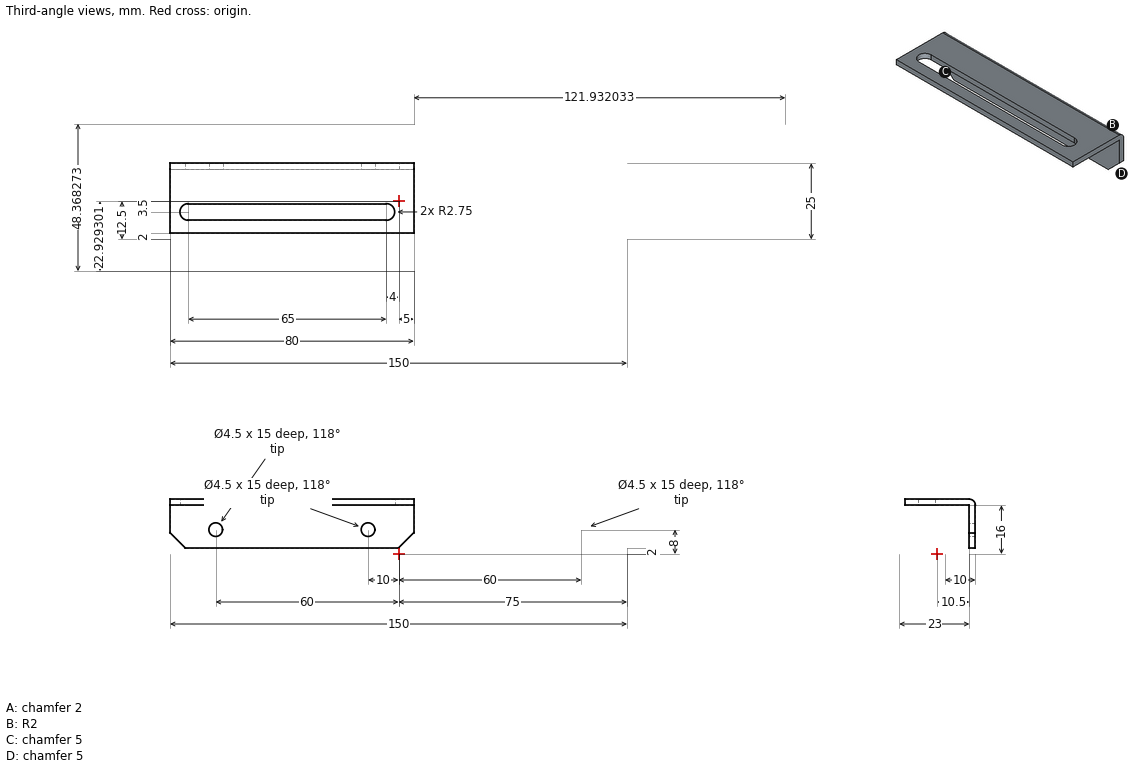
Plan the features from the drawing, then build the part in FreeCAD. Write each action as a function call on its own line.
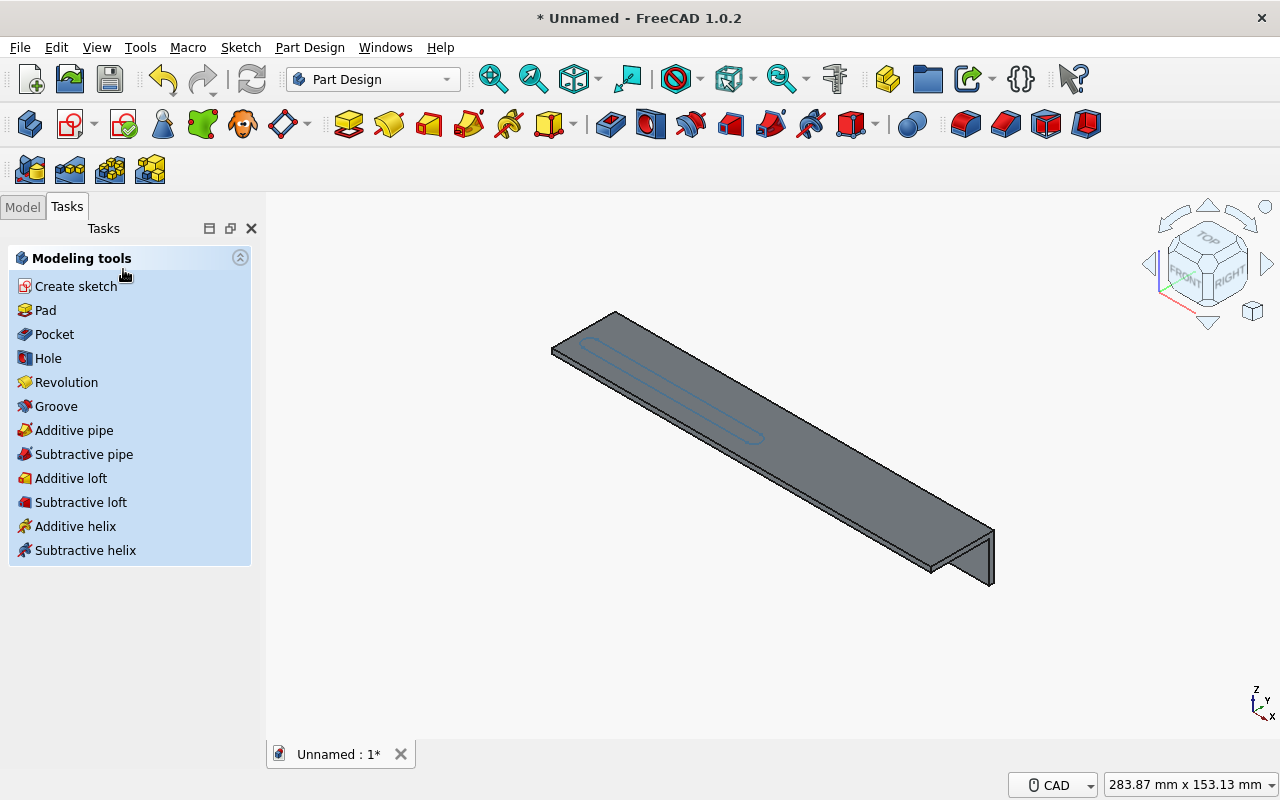
click(612, 124)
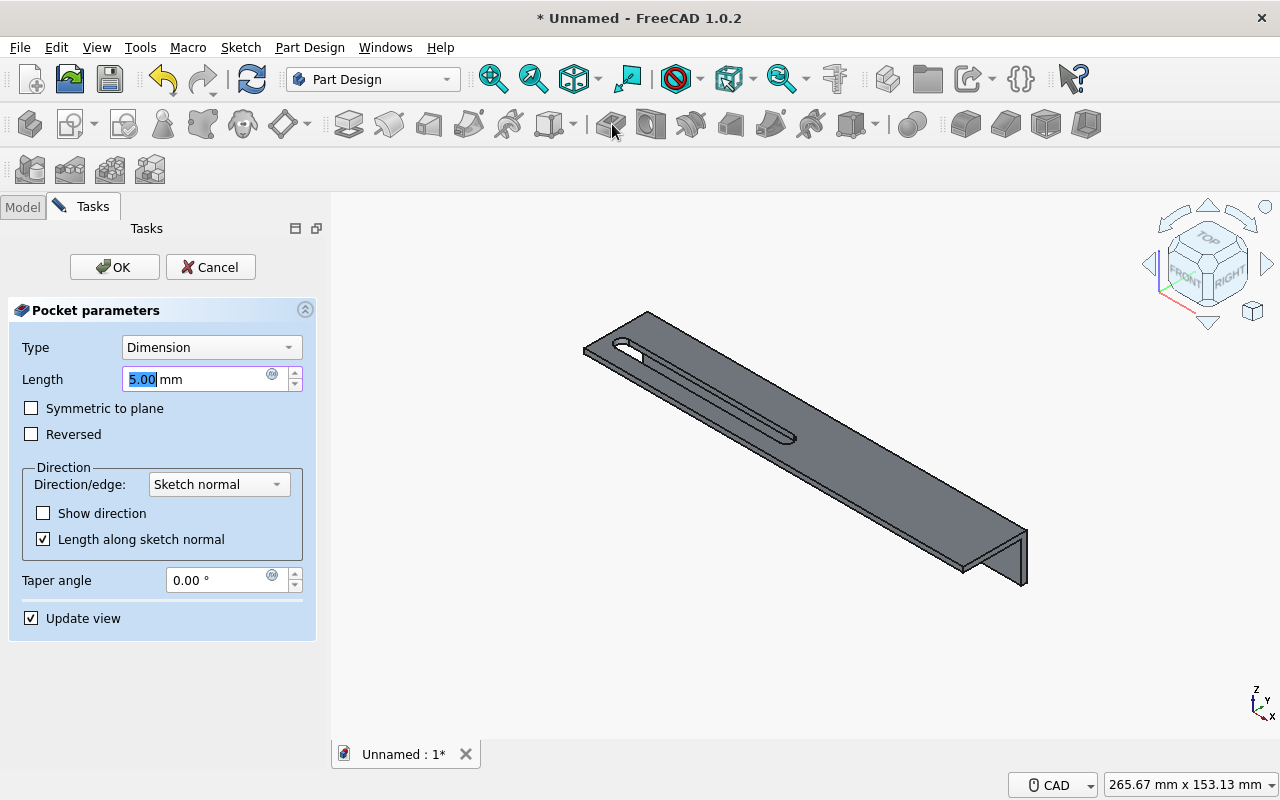
click(212, 348)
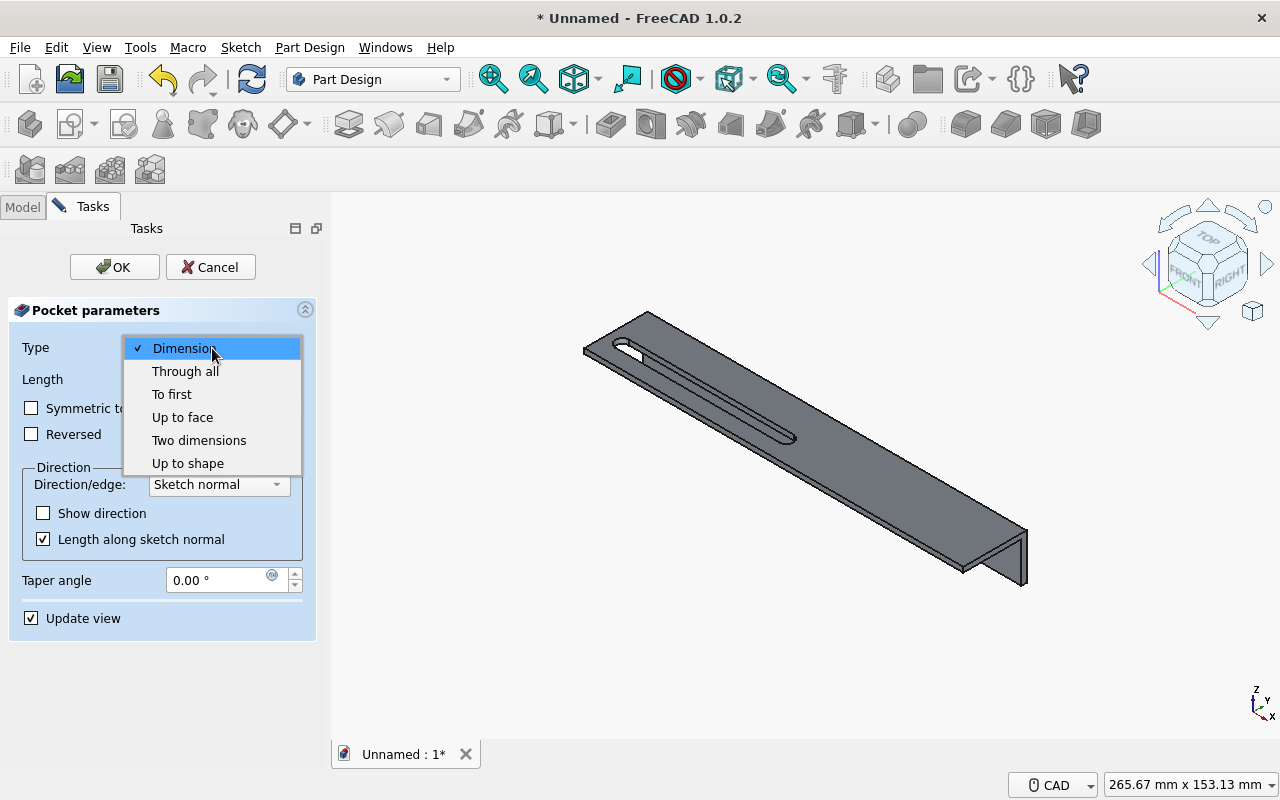
click(212, 372)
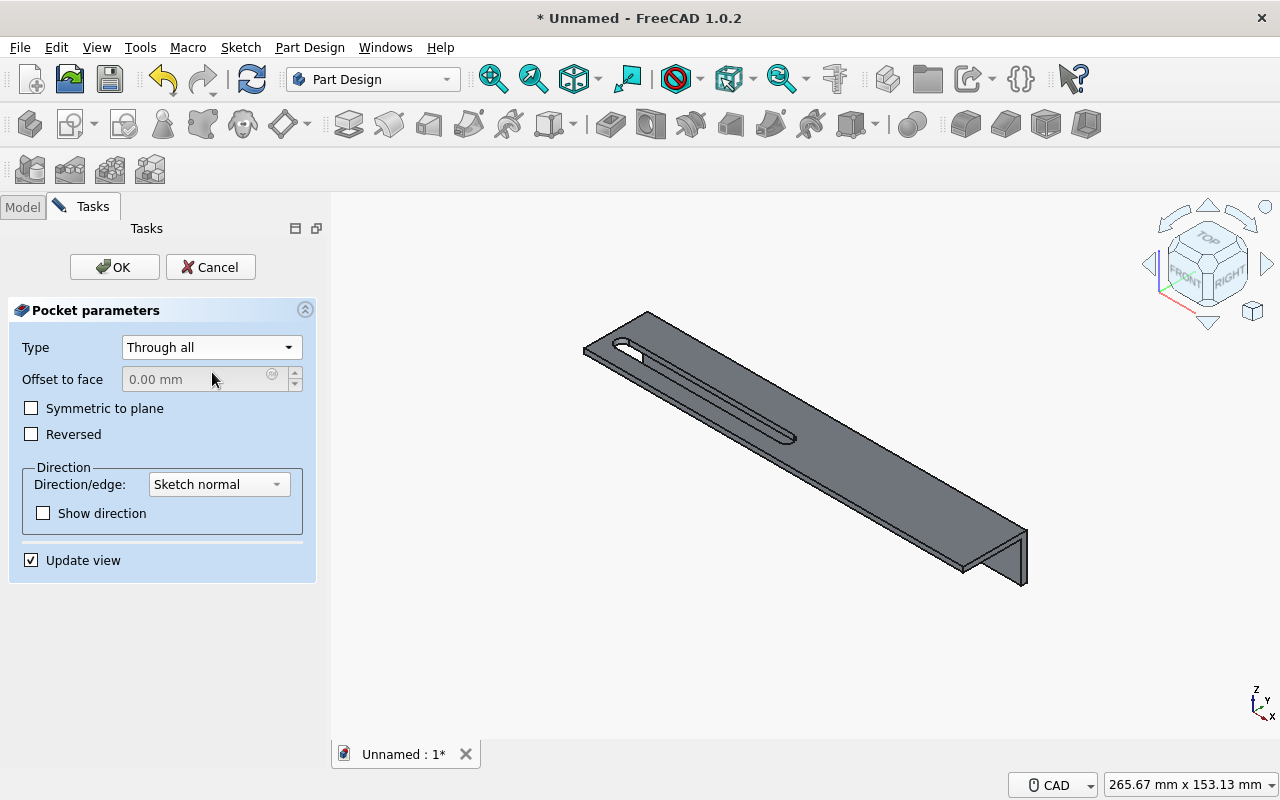
click(115, 267)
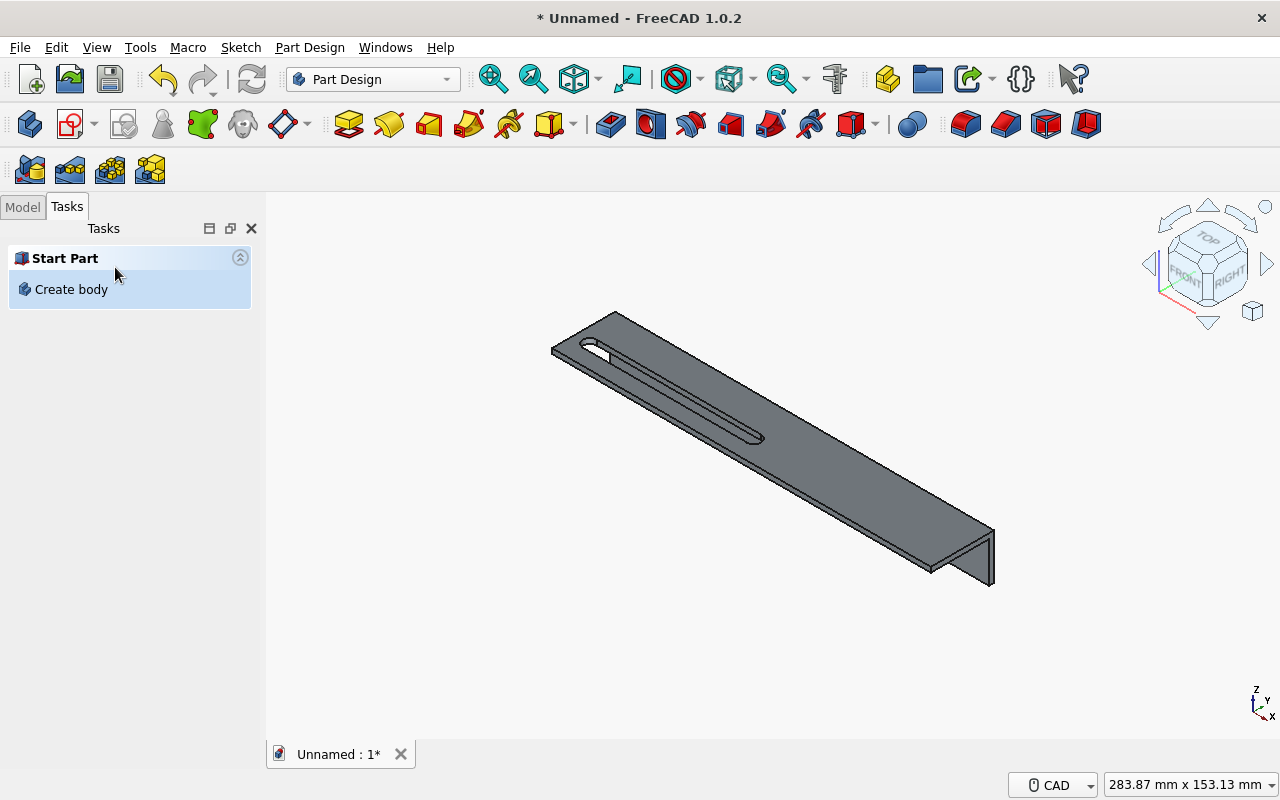
key(4)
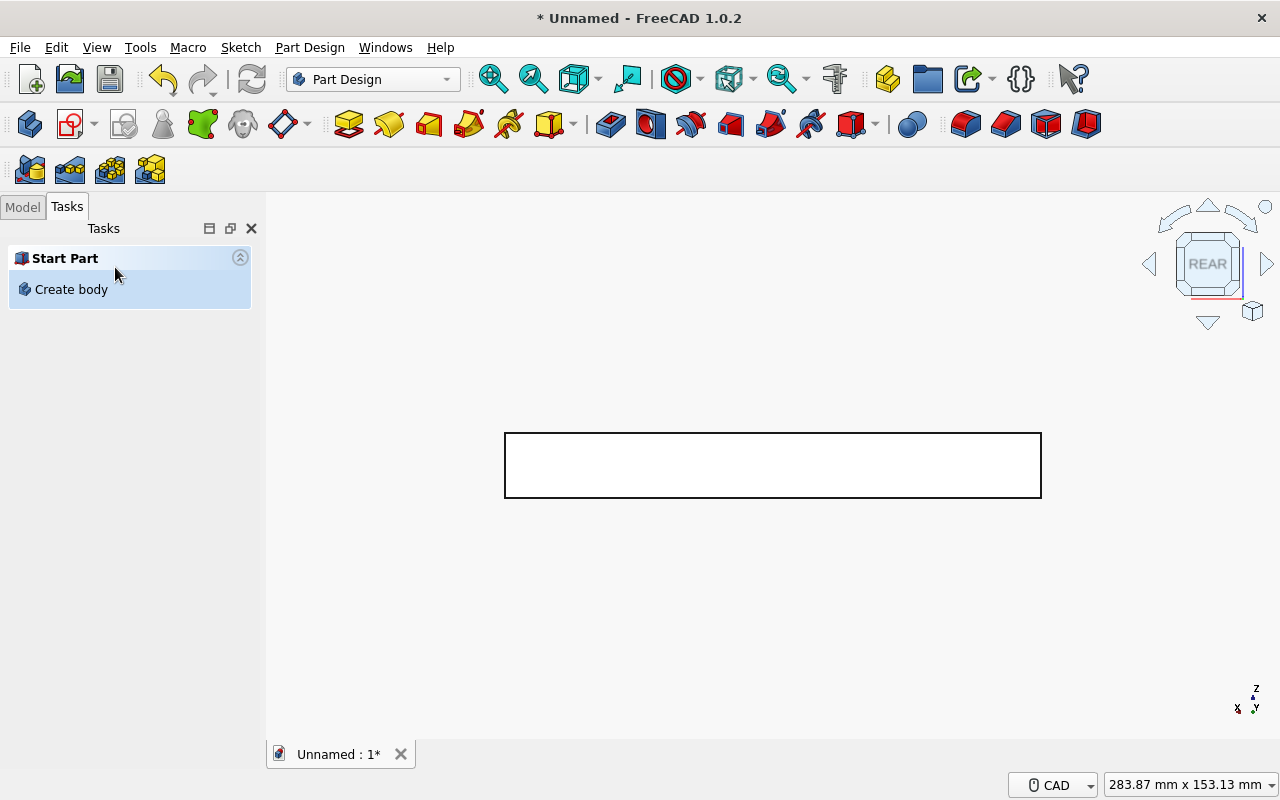
click(543, 465)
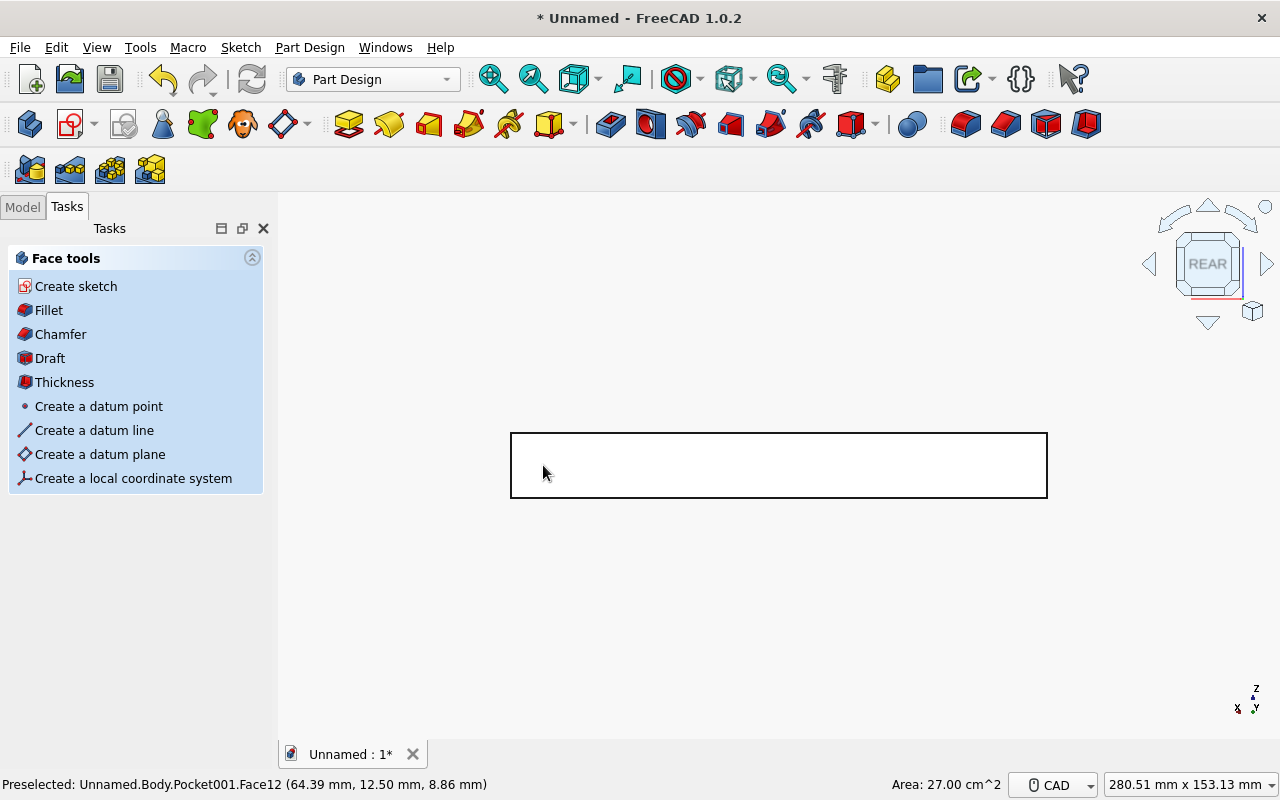
click(70, 124)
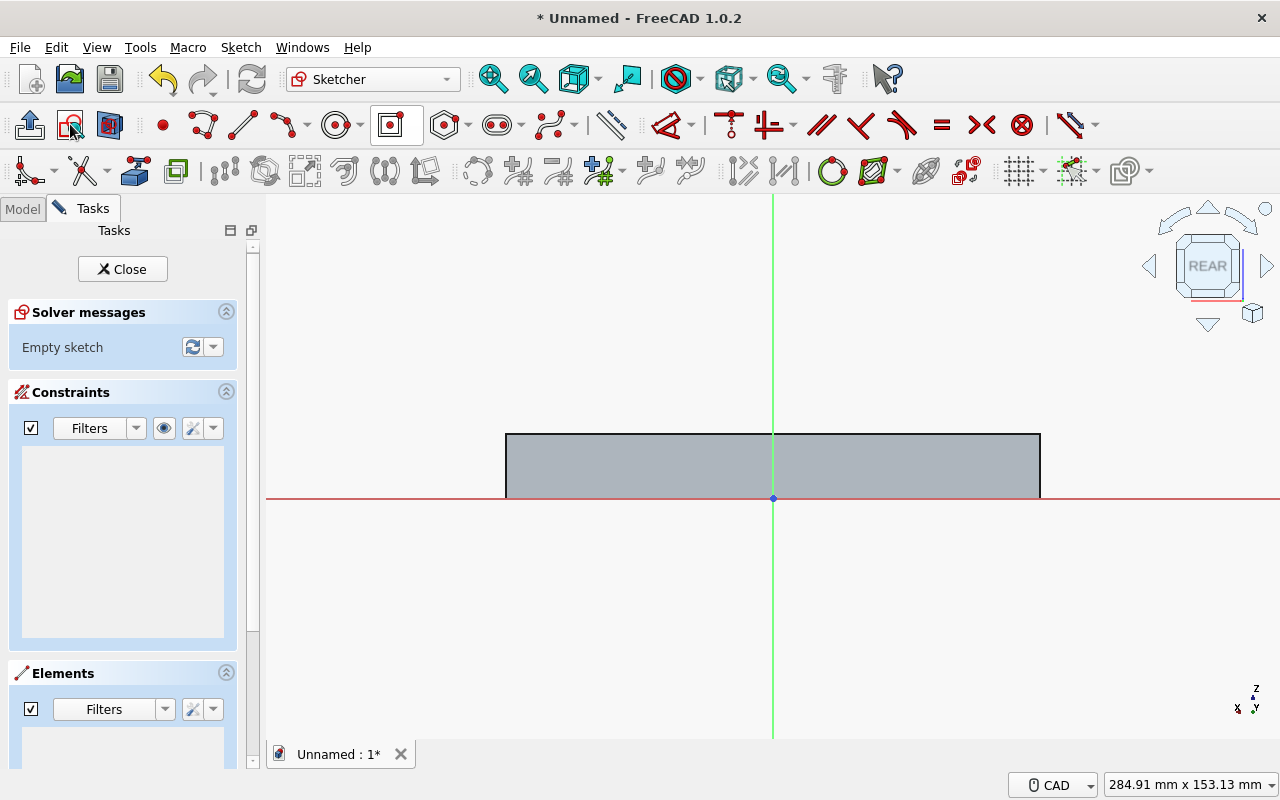
scroll(552, 470, up, 15)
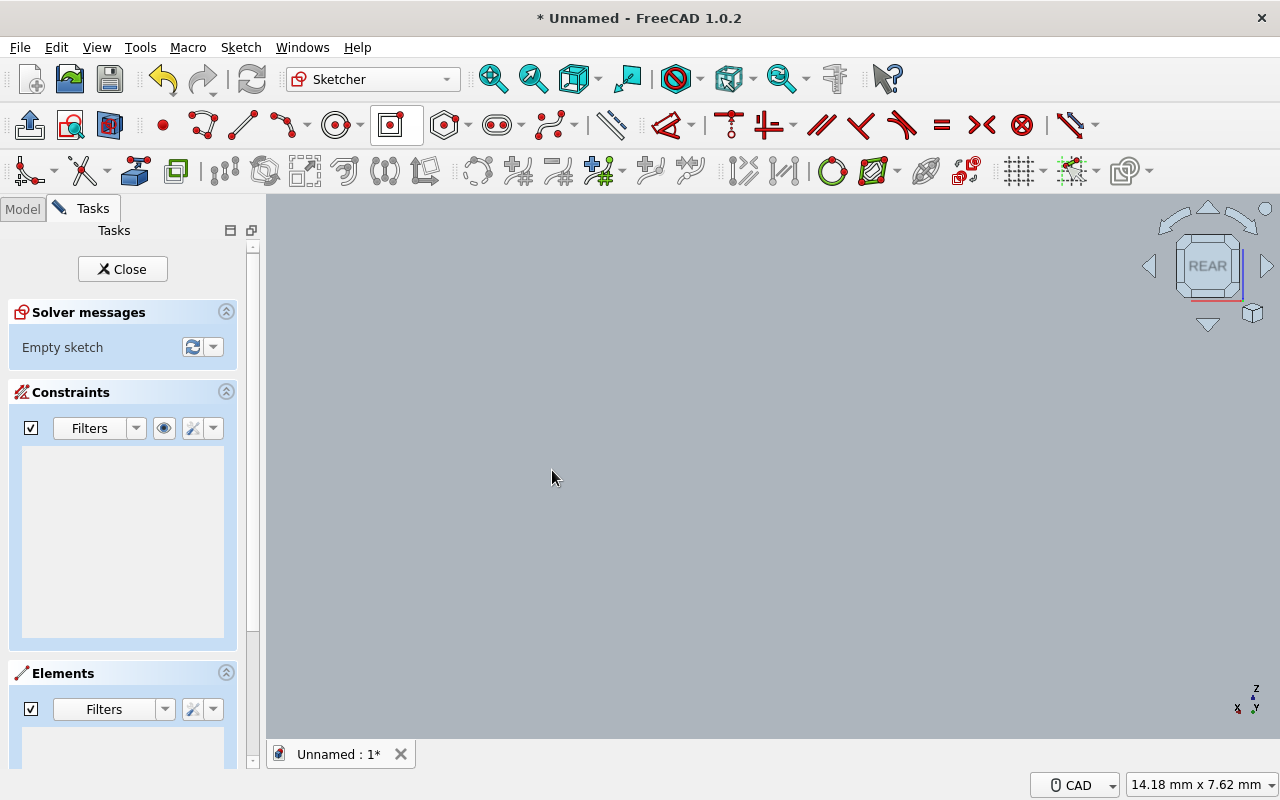
click(336, 126)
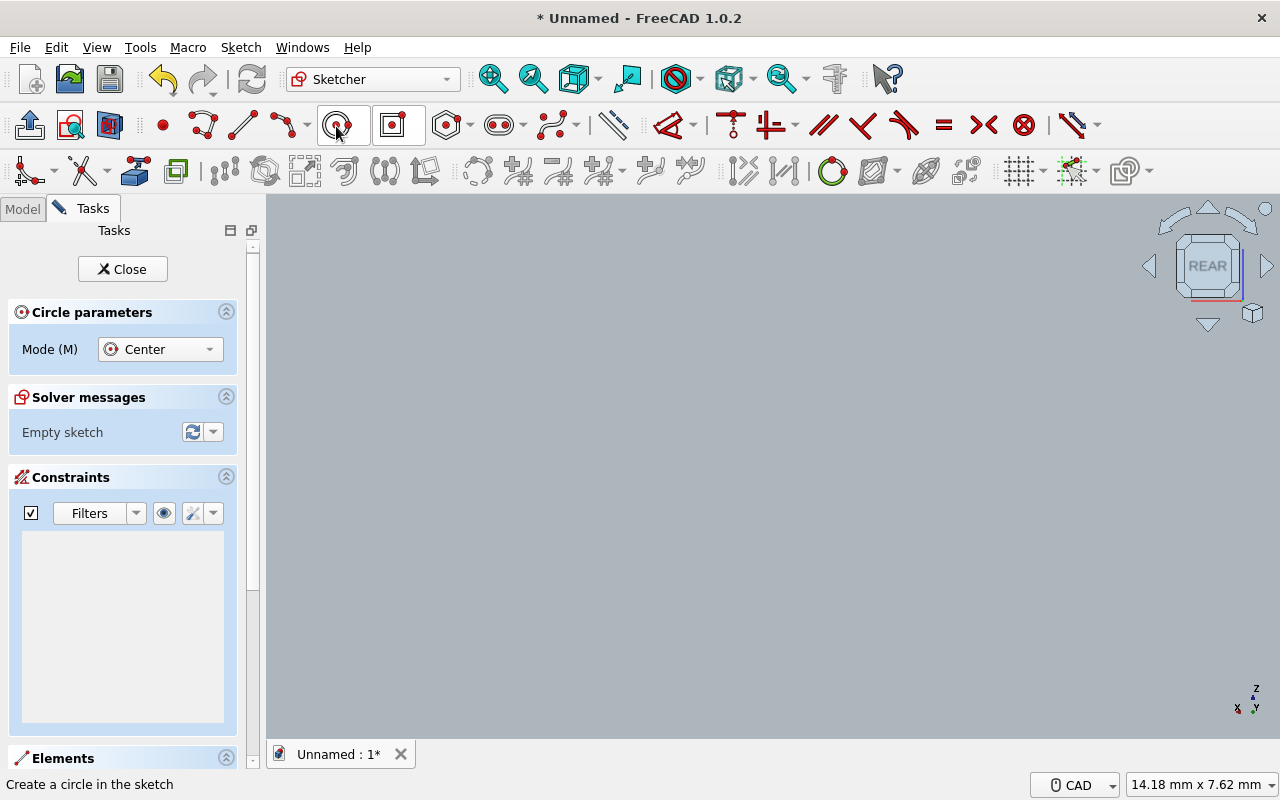
click(696, 462)
click(810, 348)
key(Escape)